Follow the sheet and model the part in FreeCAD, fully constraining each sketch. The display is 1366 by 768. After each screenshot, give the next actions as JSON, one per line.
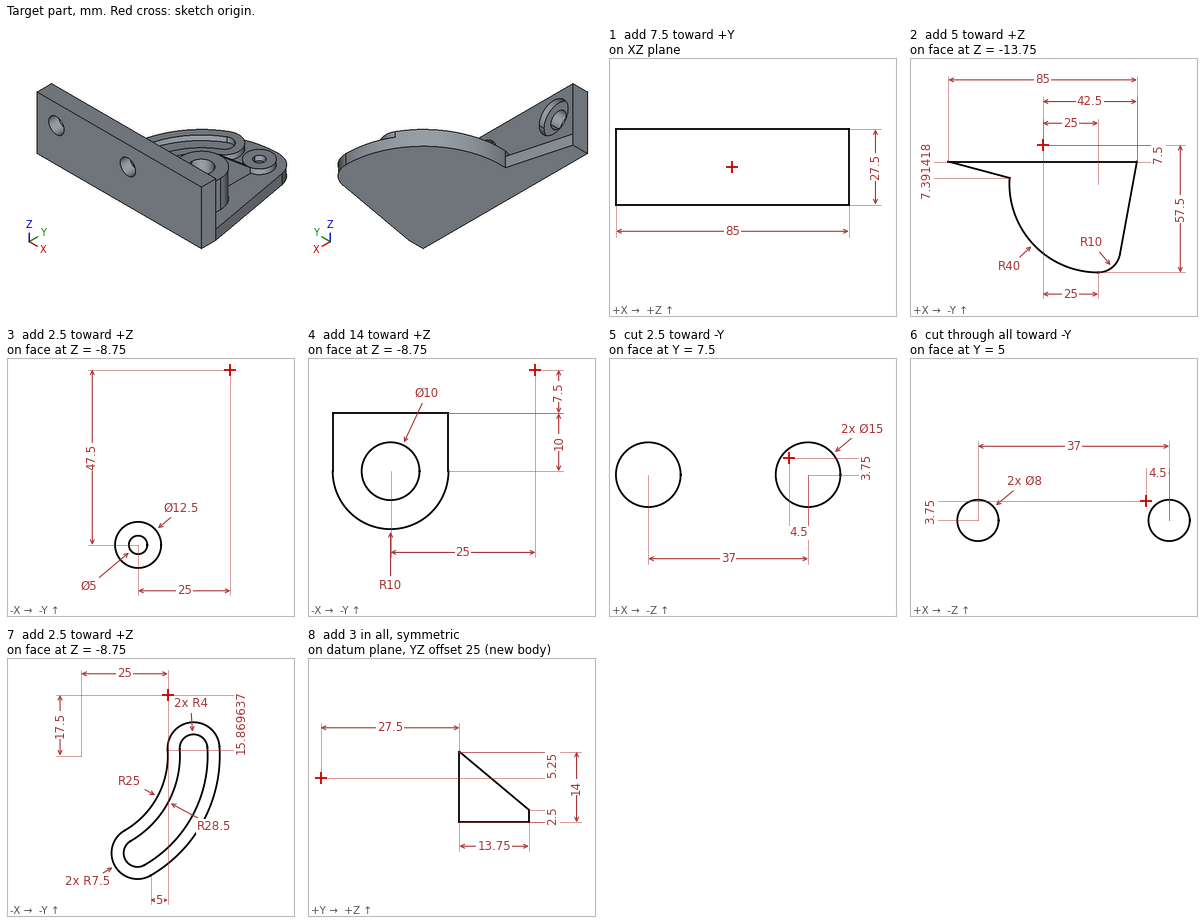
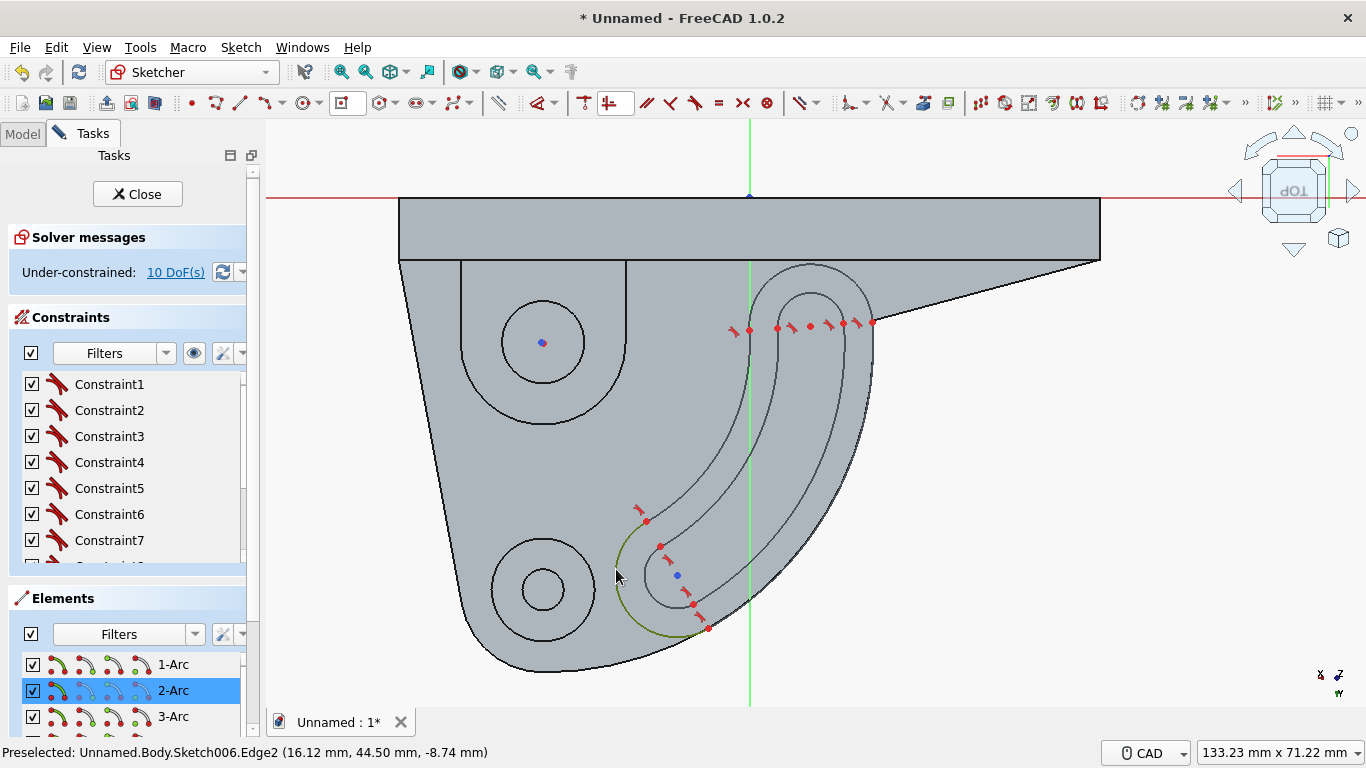
{"action": "left_click", "coordinate": [645, 572]}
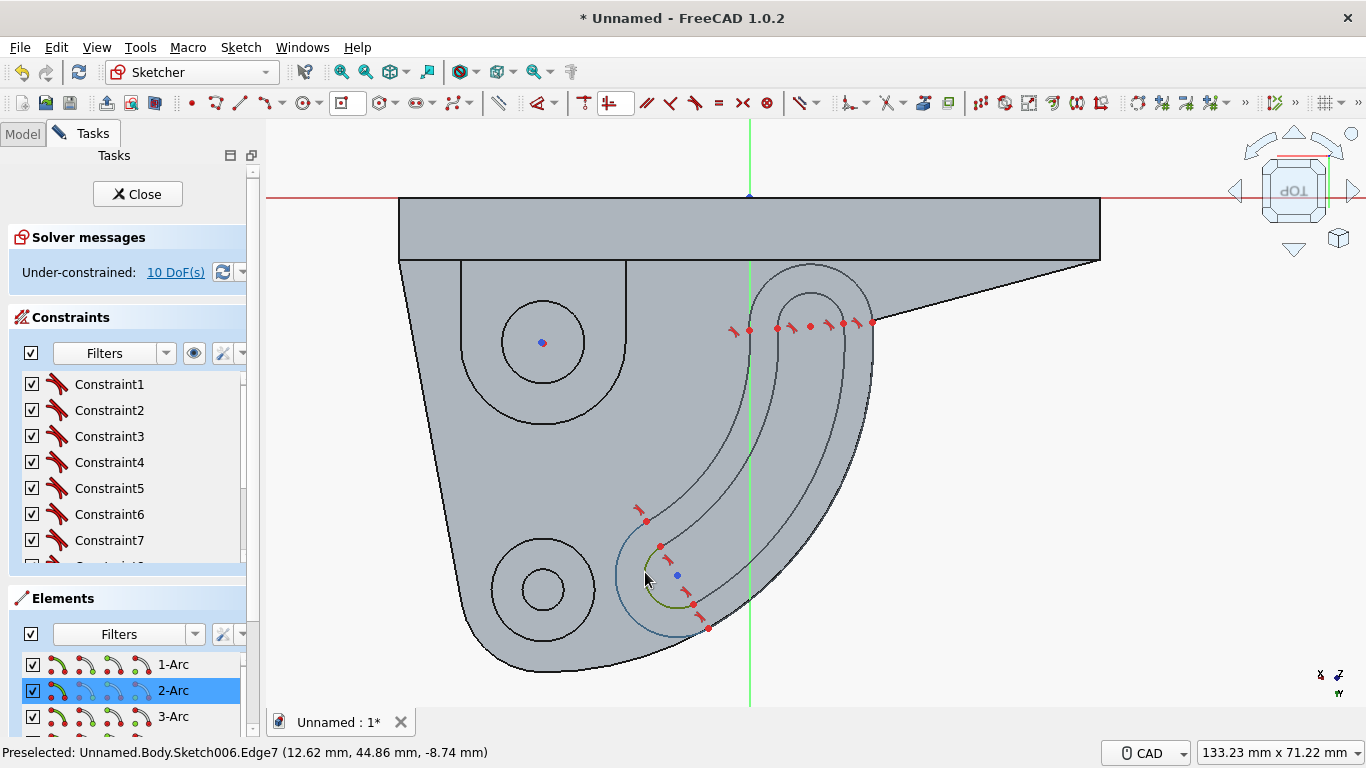
{"action": "left_click", "coordinate": [584, 104]}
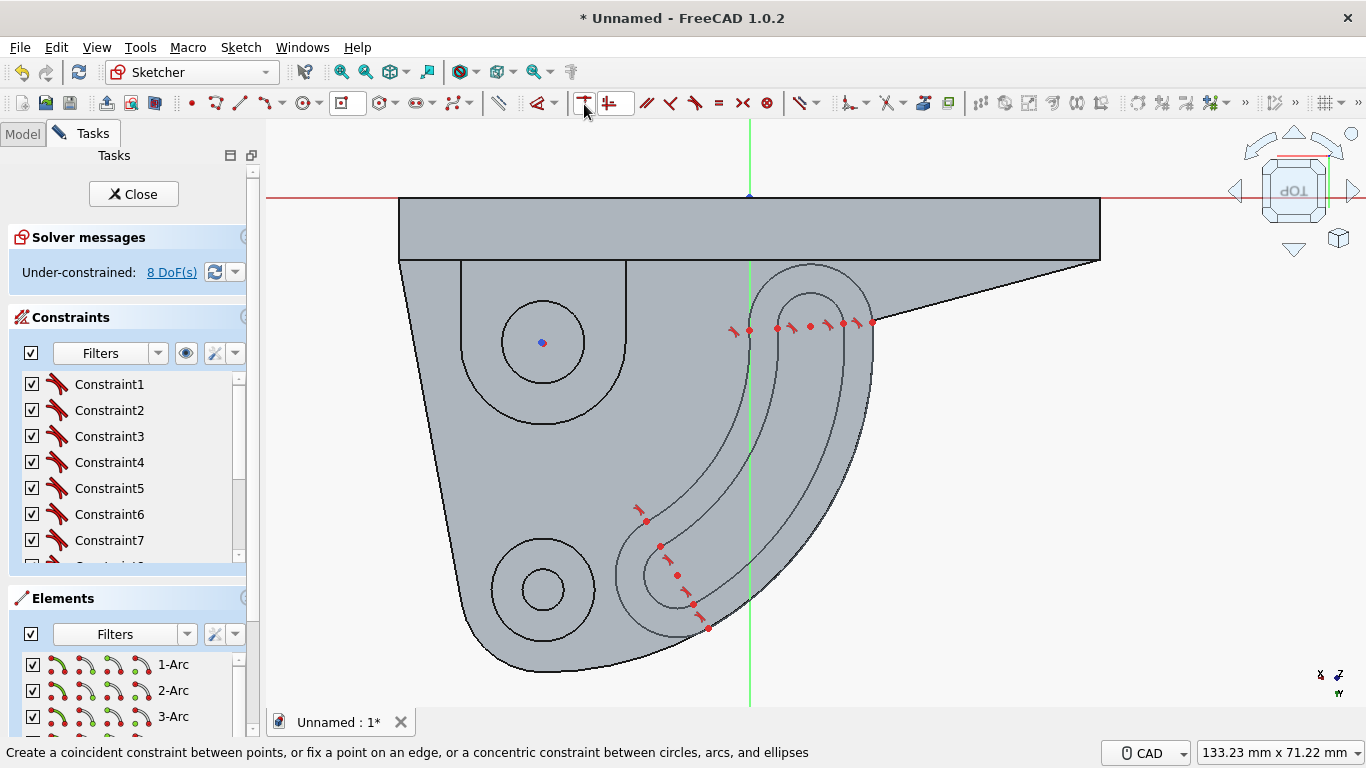
{"action": "left_click", "coordinate": [538, 104]}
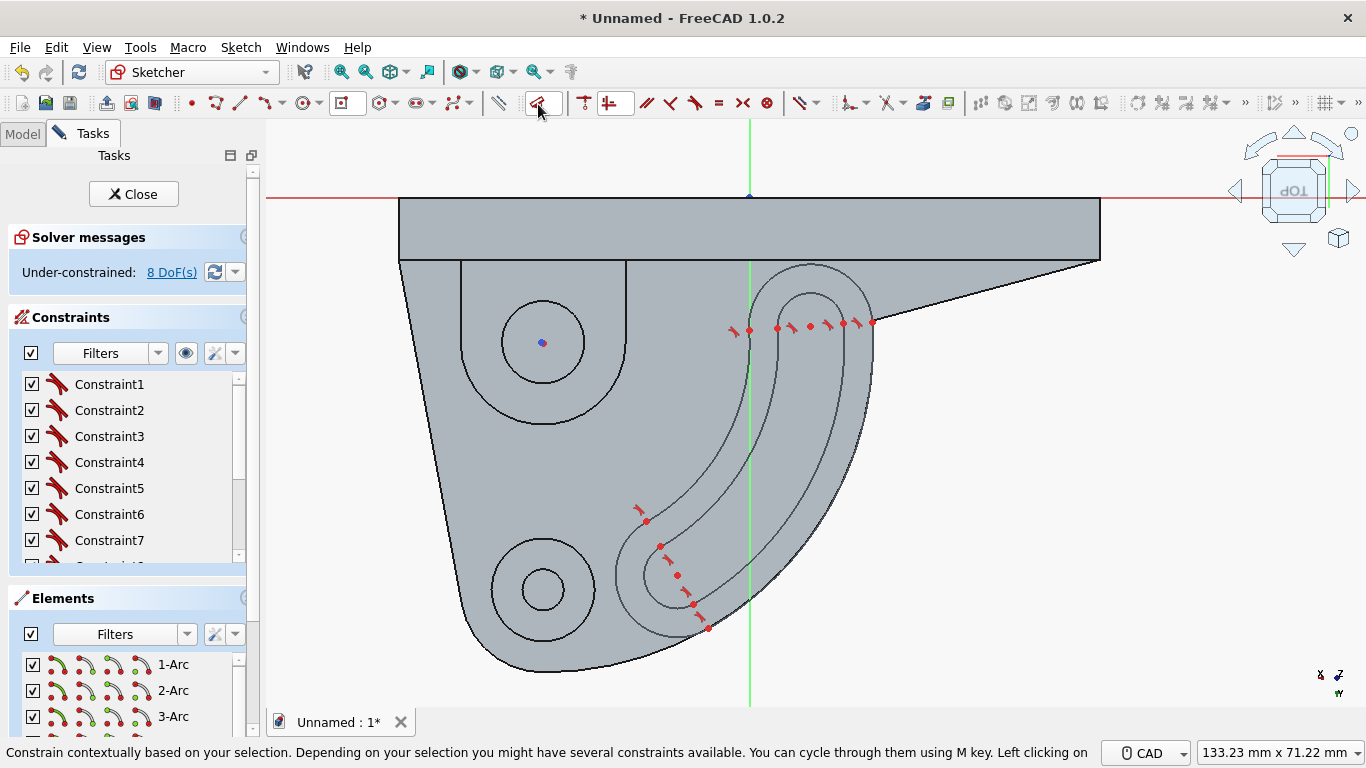
{"action": "left_click", "coordinate": [699, 478]}
{"action": "left_click", "coordinate": [510, 578]}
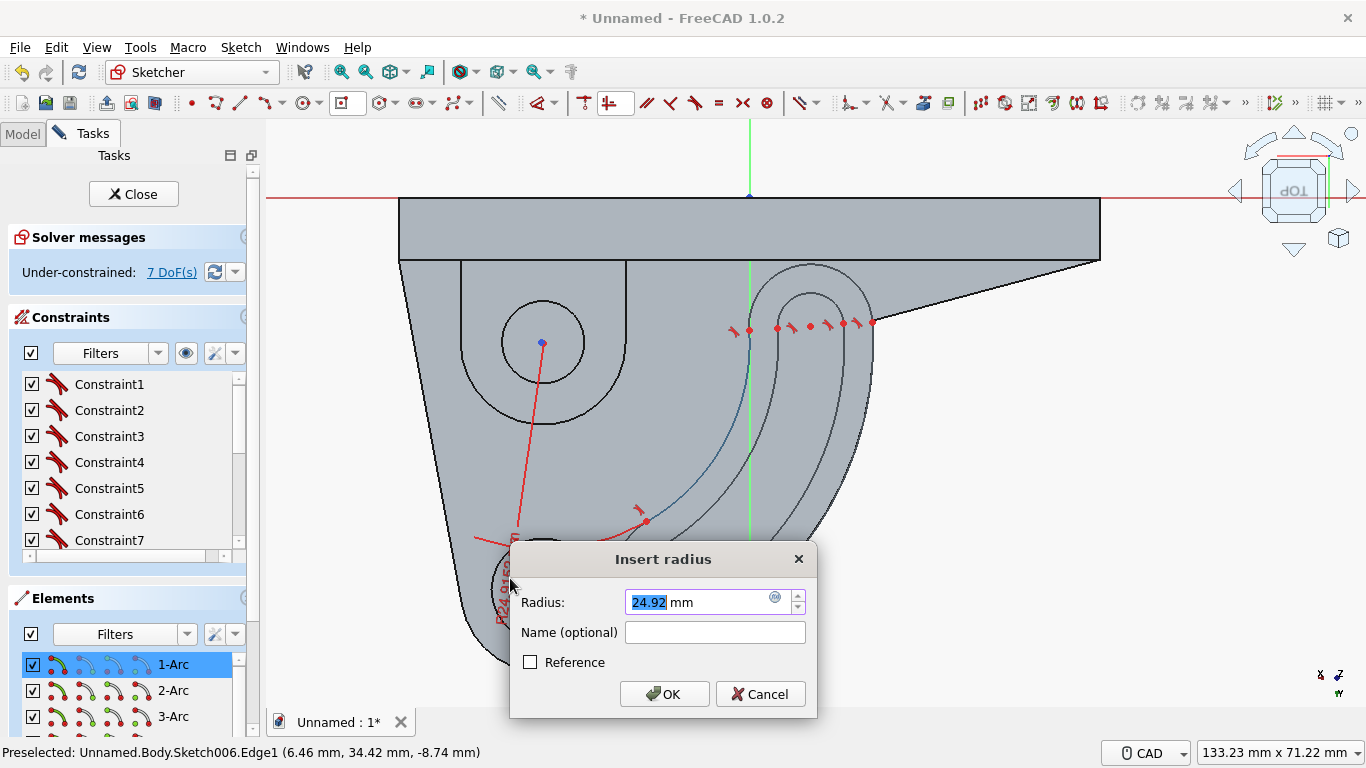
{"action": "type", "text": "25"}
{"action": "key", "text": "Return"}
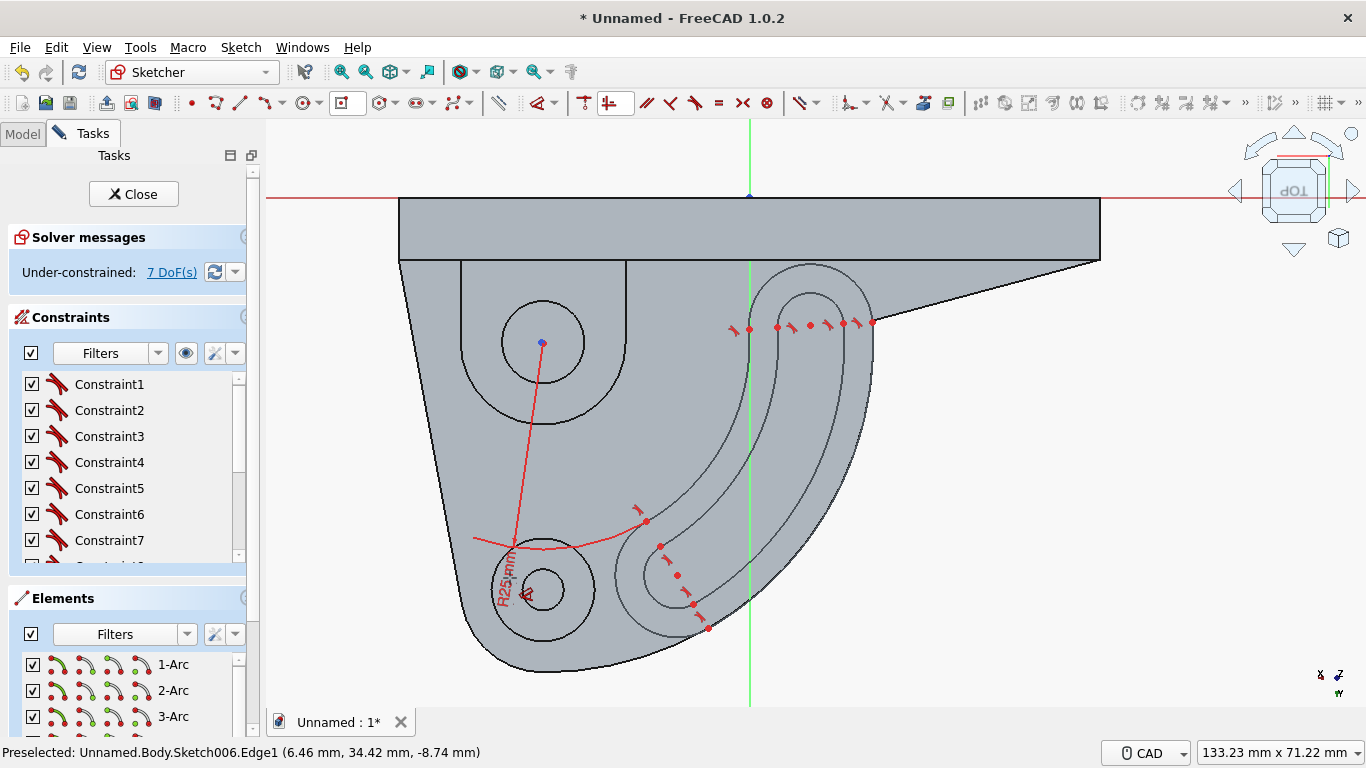
{"action": "left_click", "coordinate": [616, 569]}
{"action": "left_click", "coordinate": [584, 566]}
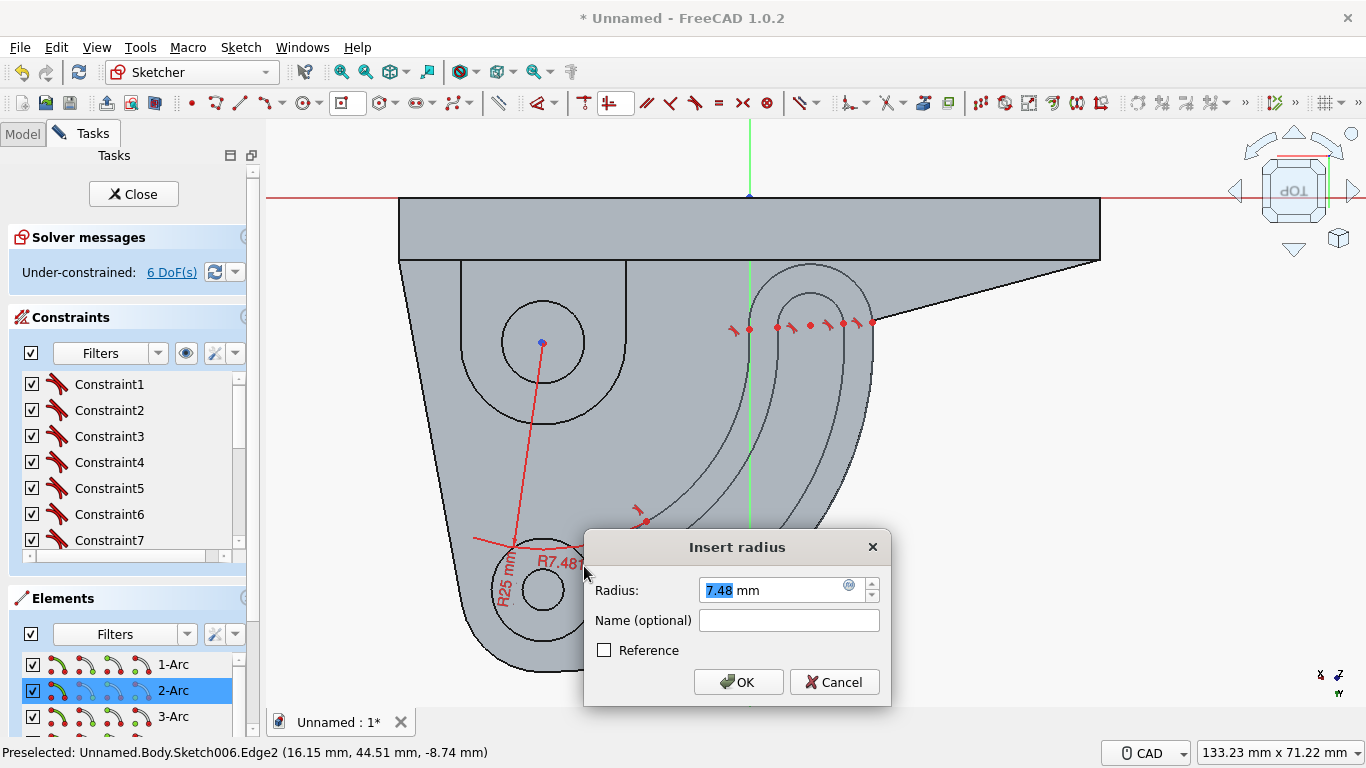
{"action": "type", "text": "7.5"}
{"action": "key", "text": "Return"}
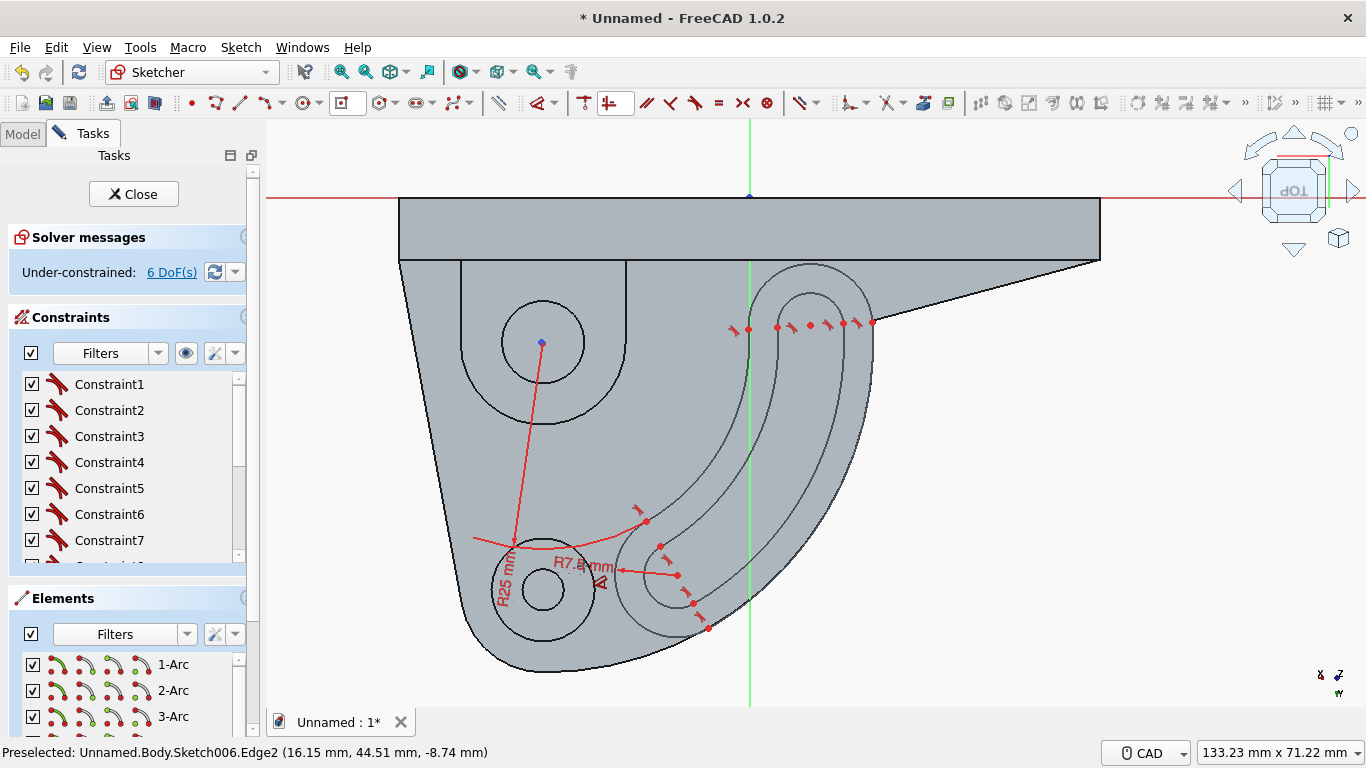
{"action": "left_click", "coordinate": [828, 298]}
{"action": "left_click", "coordinate": [857, 251]}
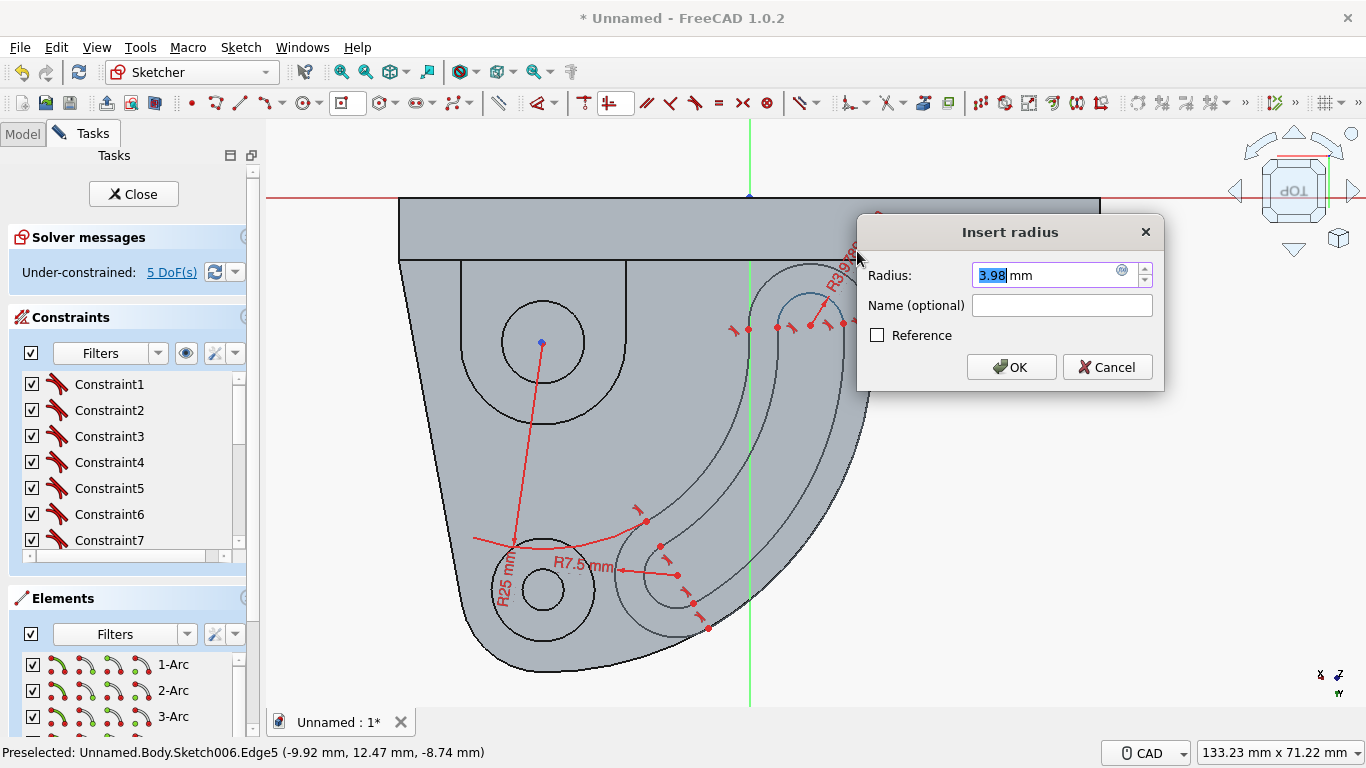
{"action": "type", "text": "4"}
{"action": "key", "text": "Return"}